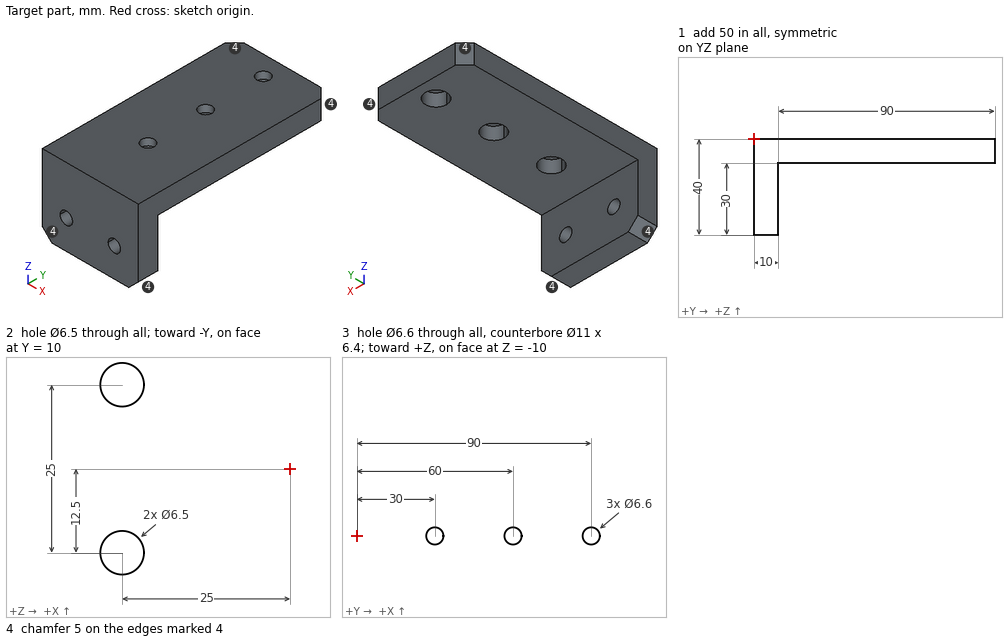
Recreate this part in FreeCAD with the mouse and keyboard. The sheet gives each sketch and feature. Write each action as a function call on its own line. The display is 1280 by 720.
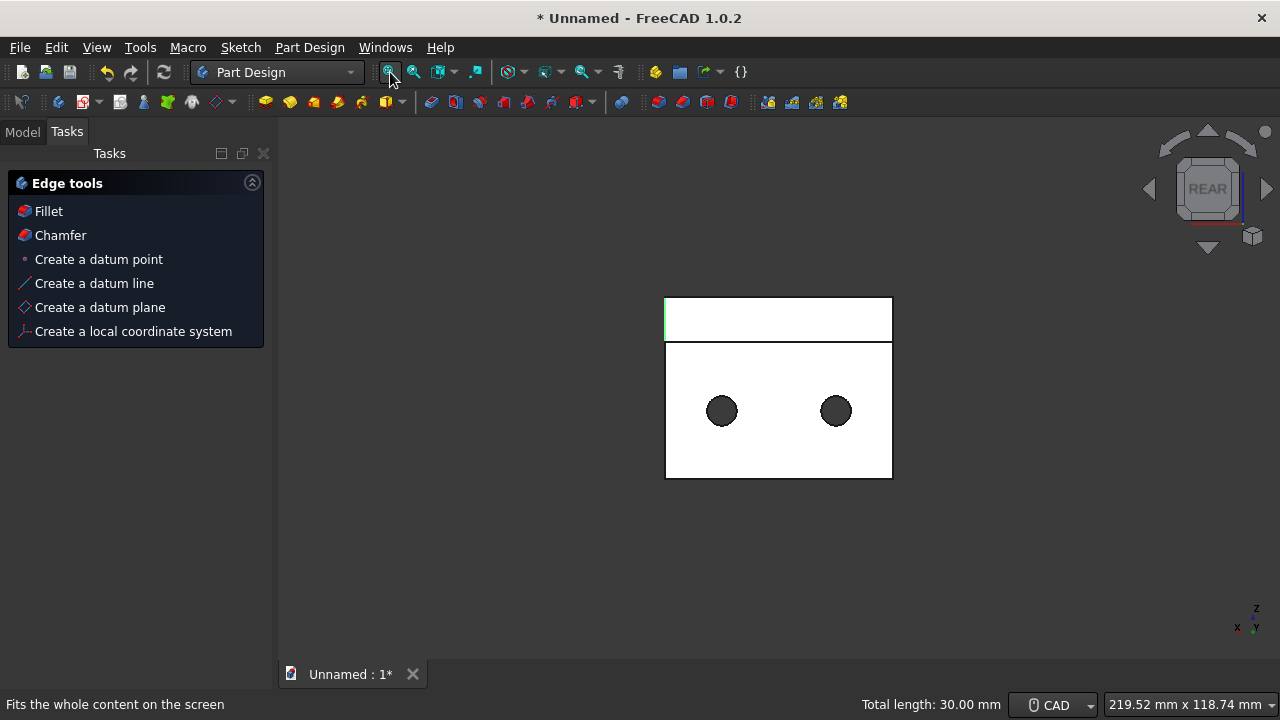
click(893, 319, ctrl)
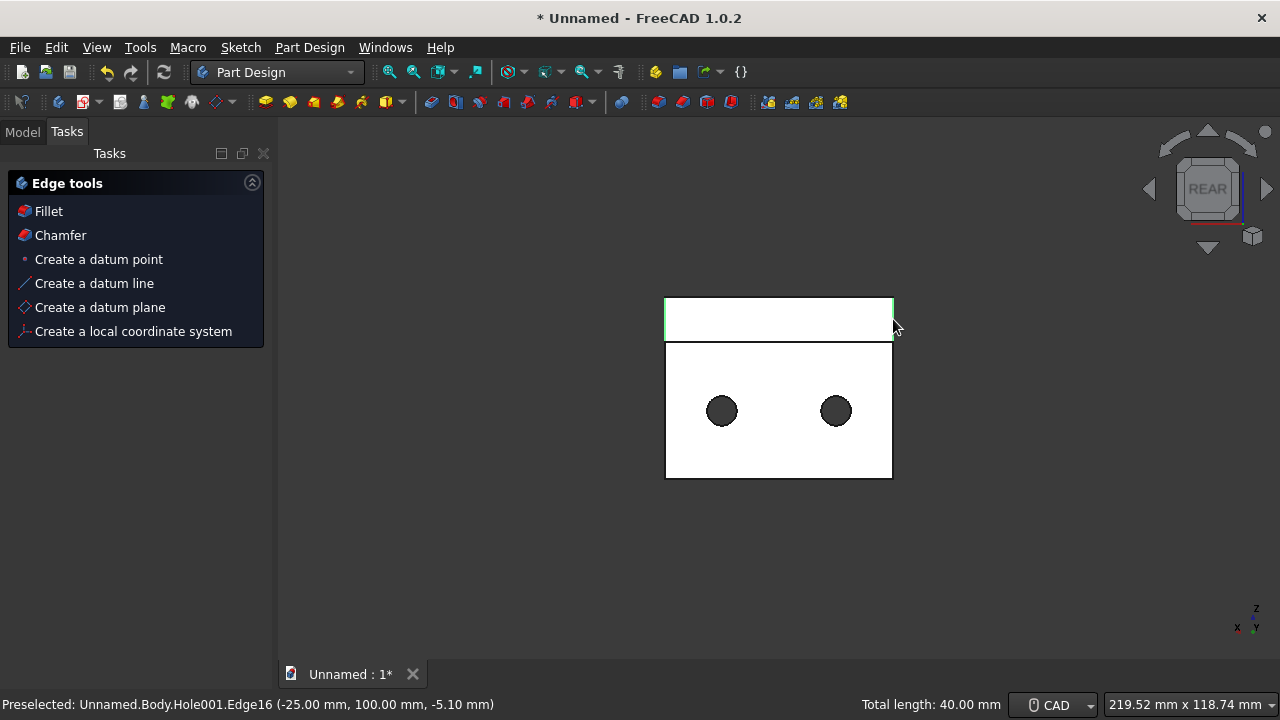
click(684, 102)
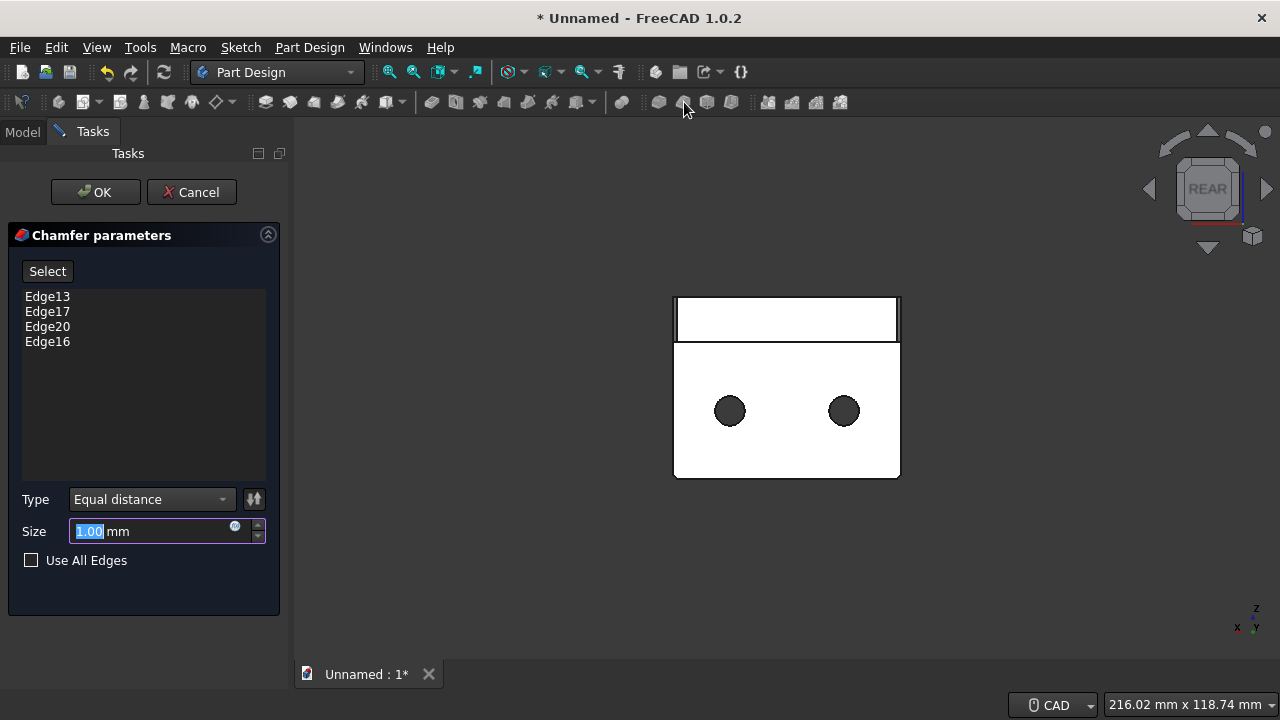
text(5)
key(Tab)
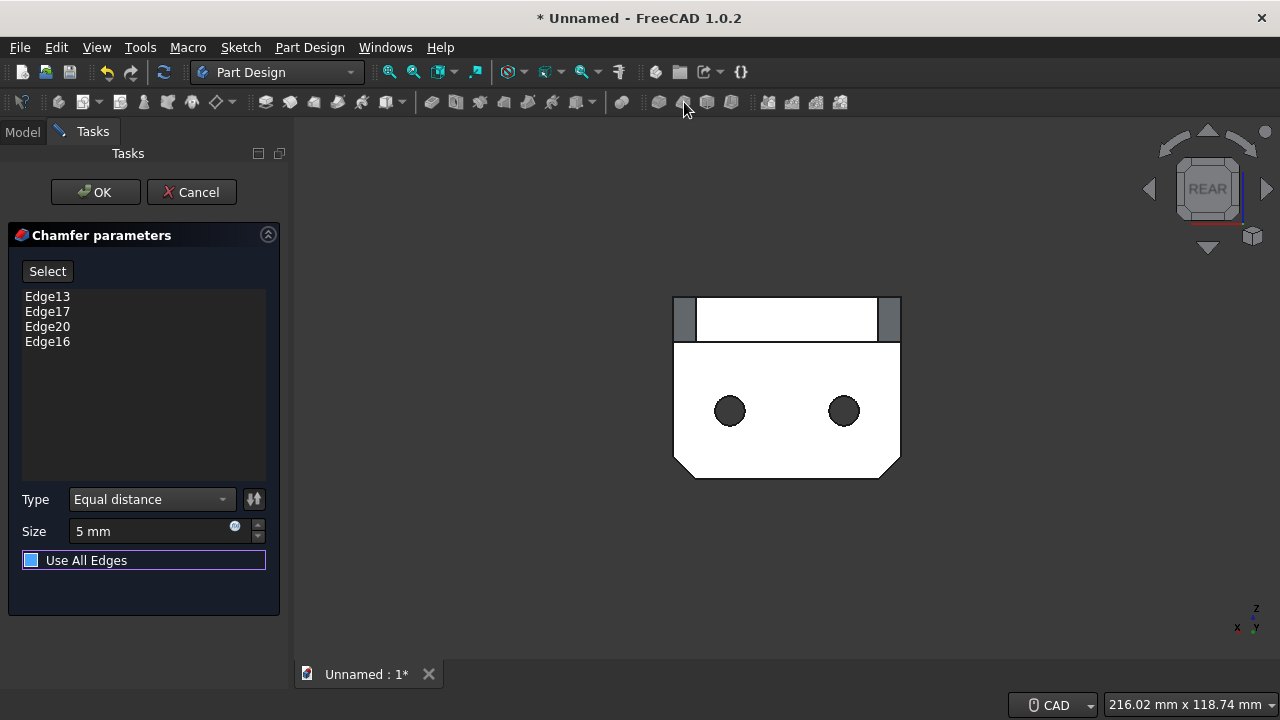
click(96, 192)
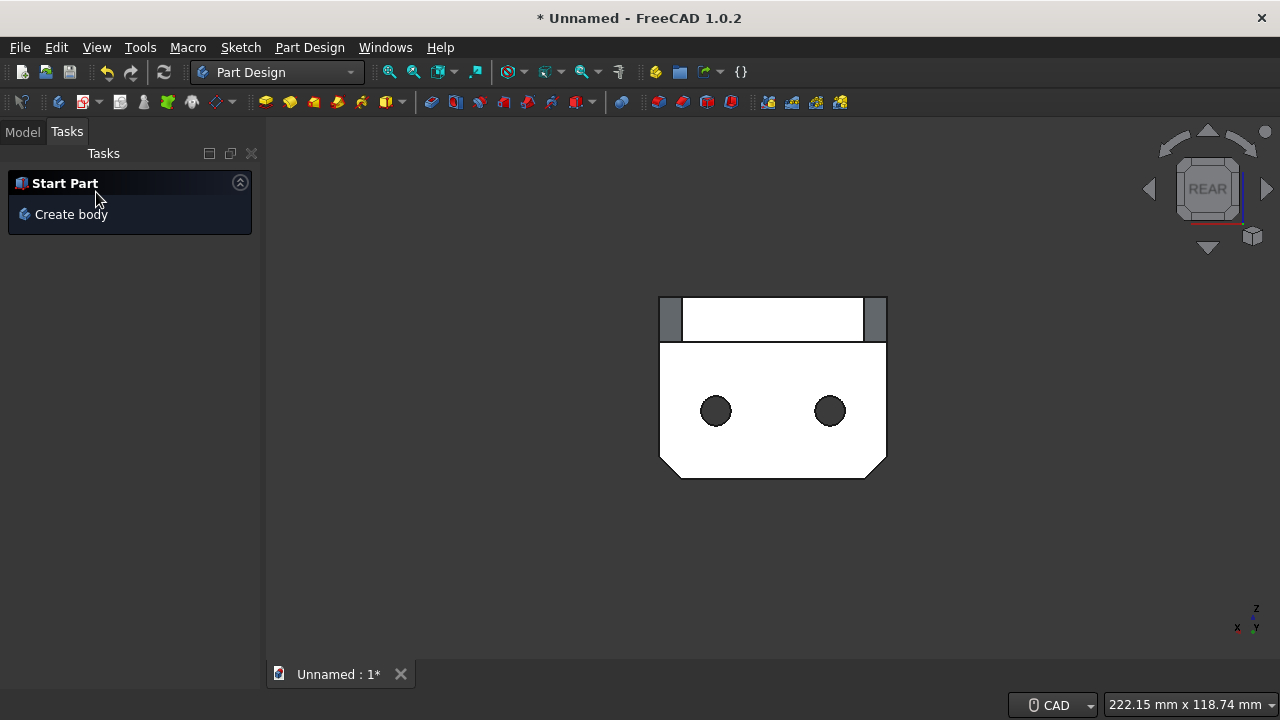
key(0)